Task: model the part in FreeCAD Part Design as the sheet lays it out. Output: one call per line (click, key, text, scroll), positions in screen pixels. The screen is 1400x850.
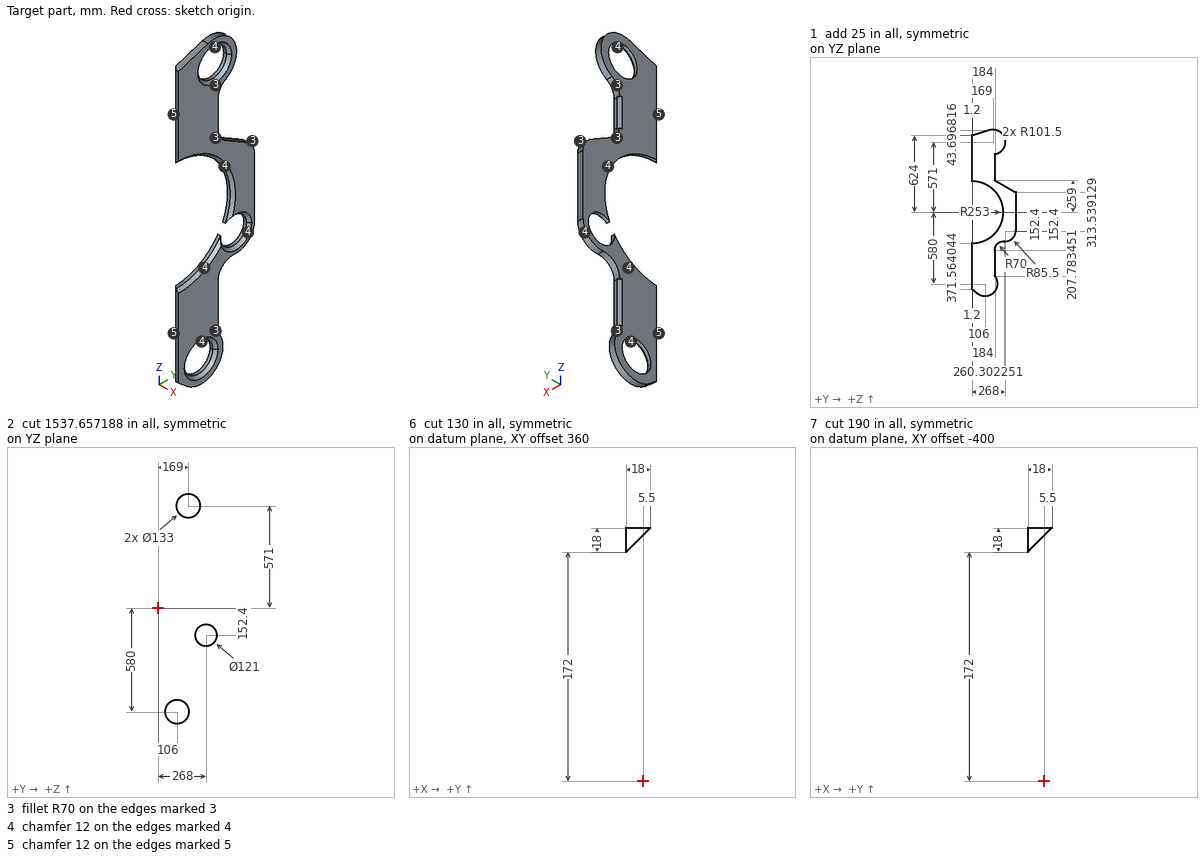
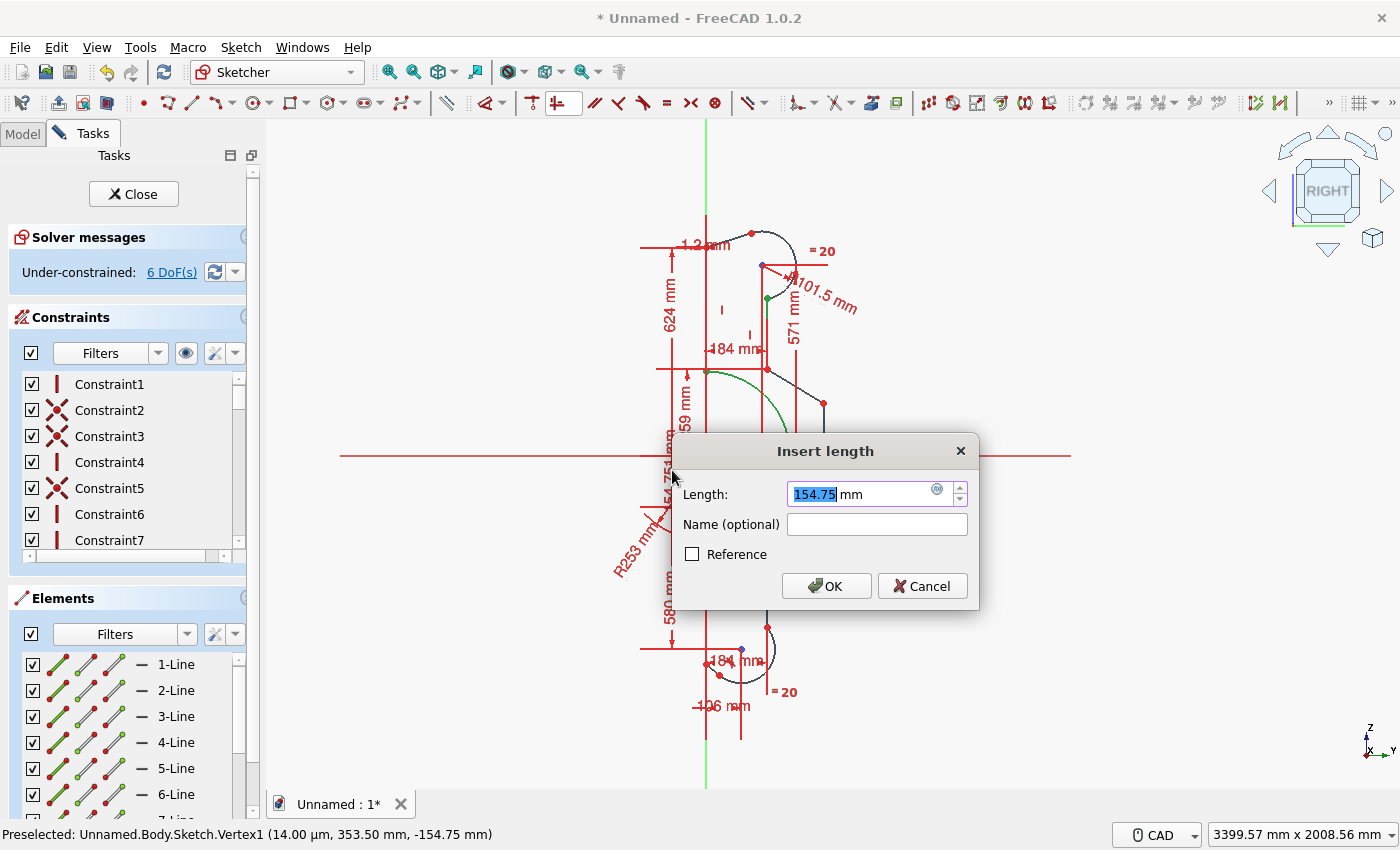
text(152.4)
key(Return)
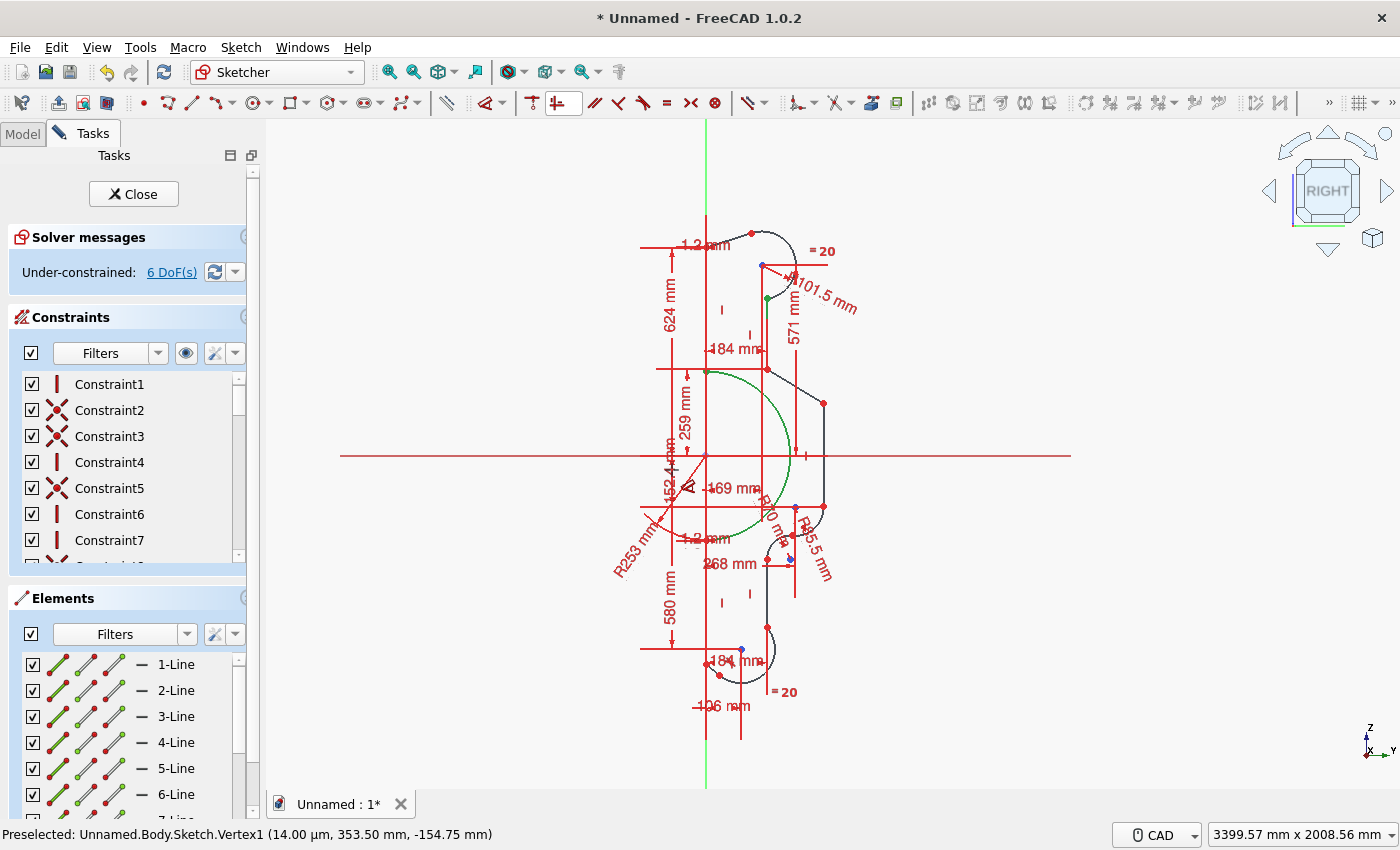
click(795, 507)
click(648, 493)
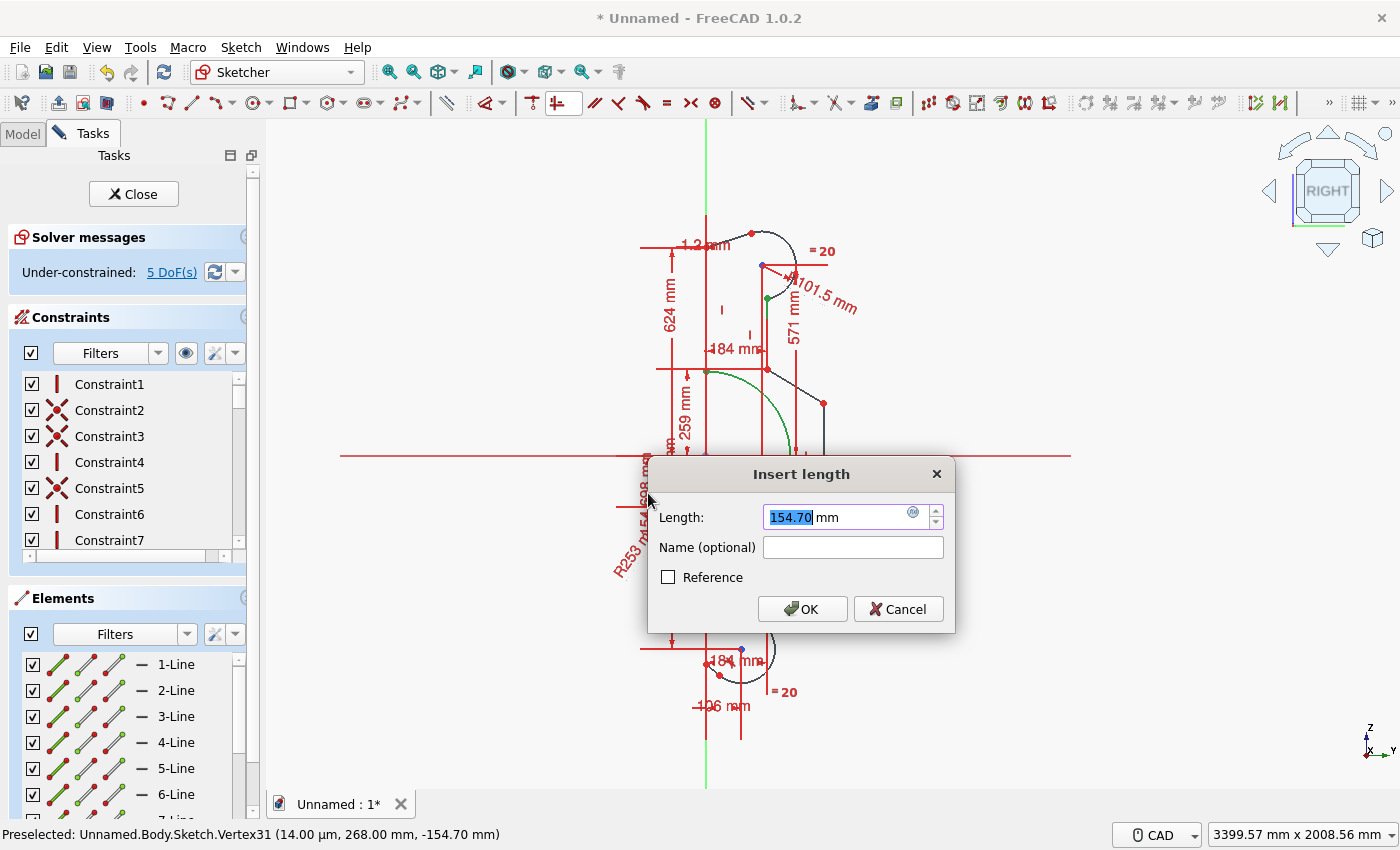
text(152.4)
key(Return)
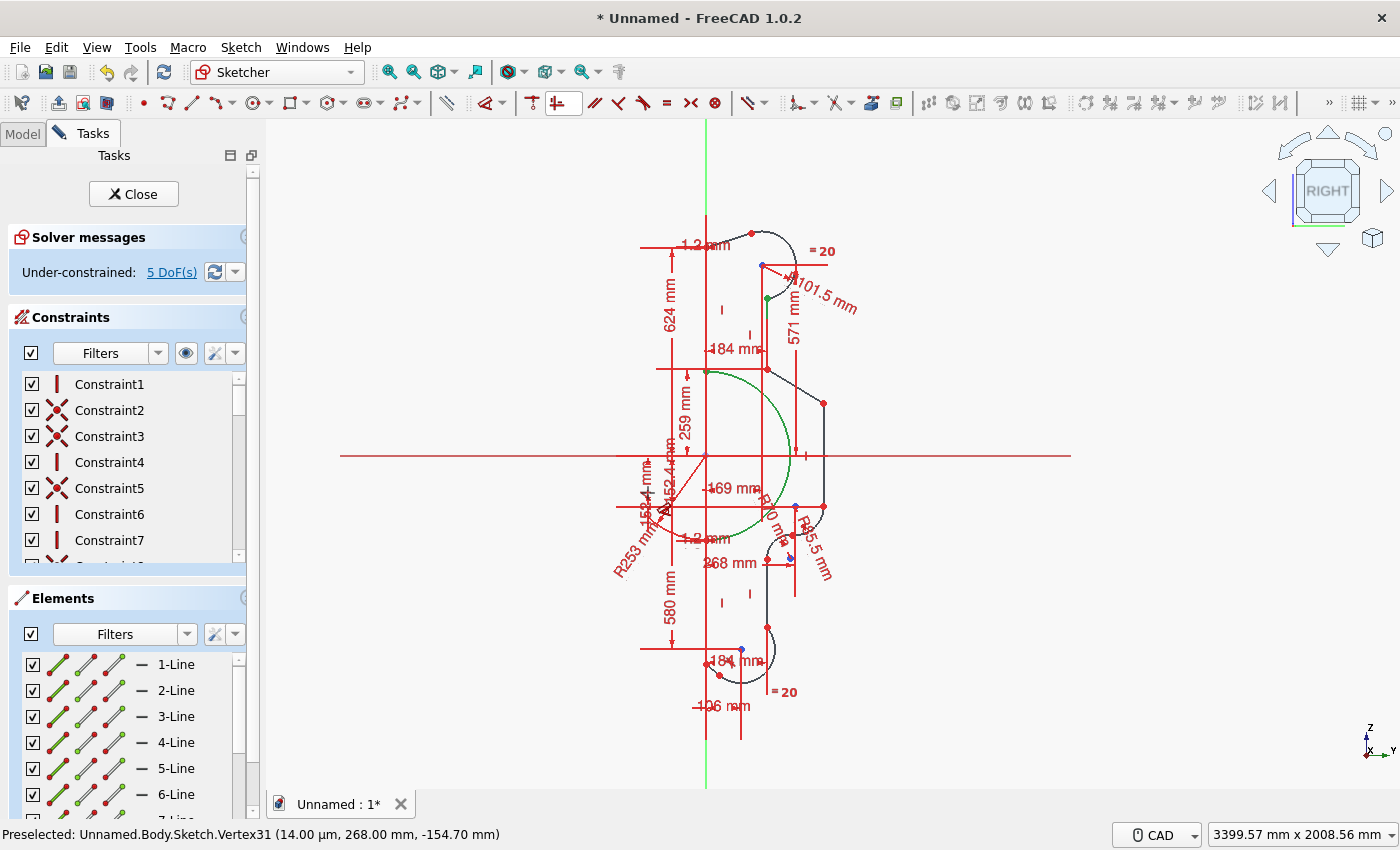
click(824, 476)
click(858, 431)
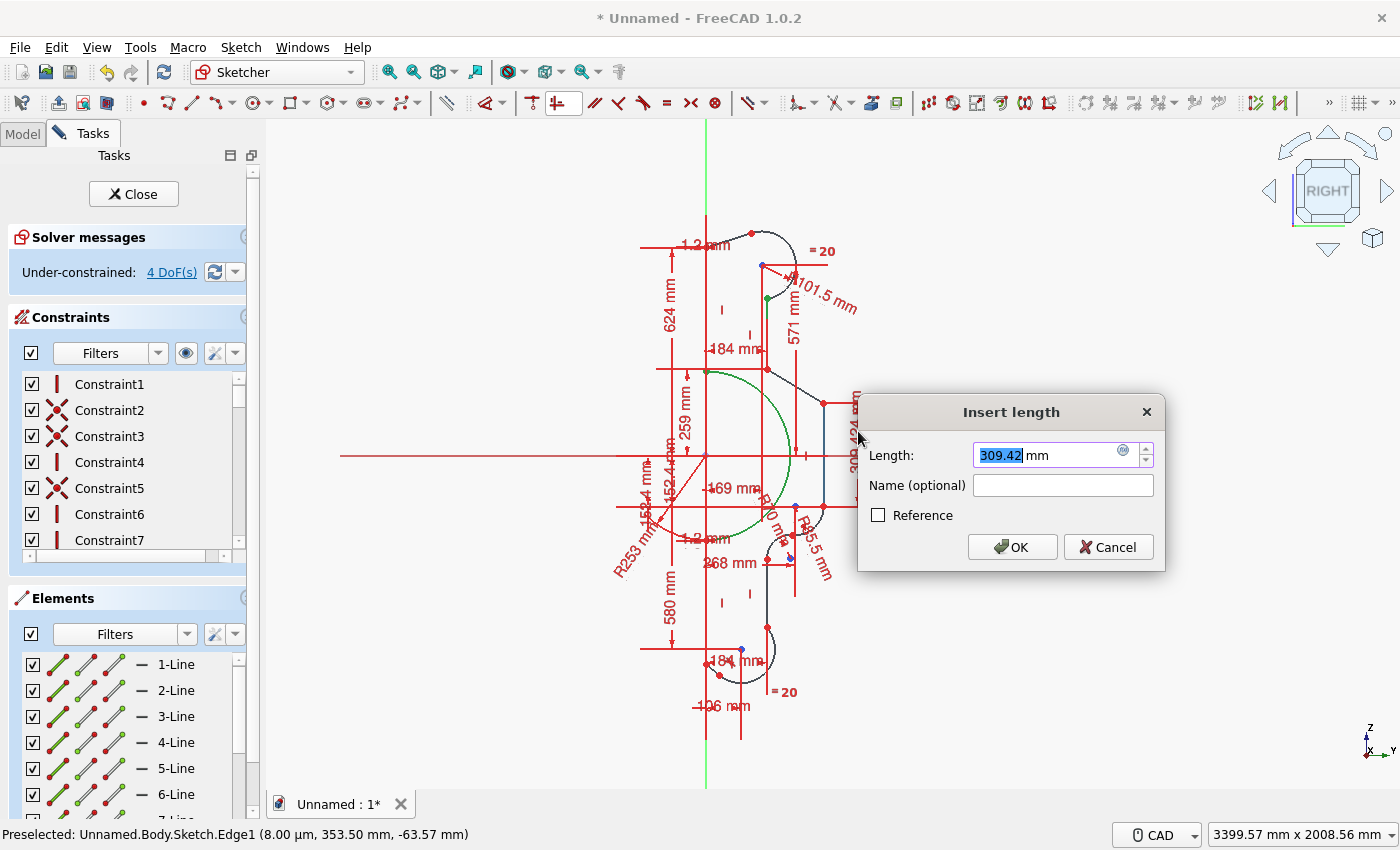
text(313.539129)
key(Return)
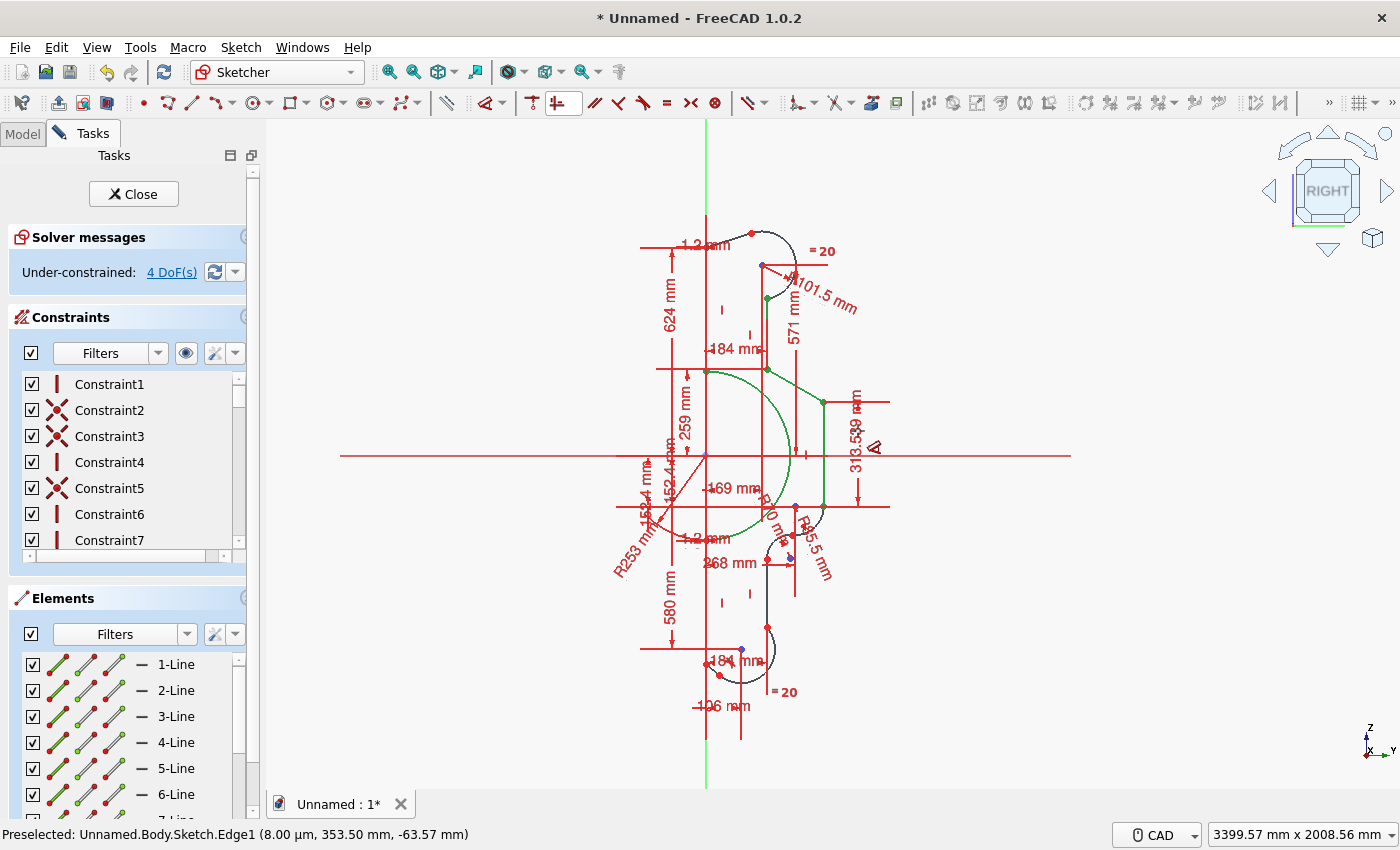
click(706, 577)
click(672, 631)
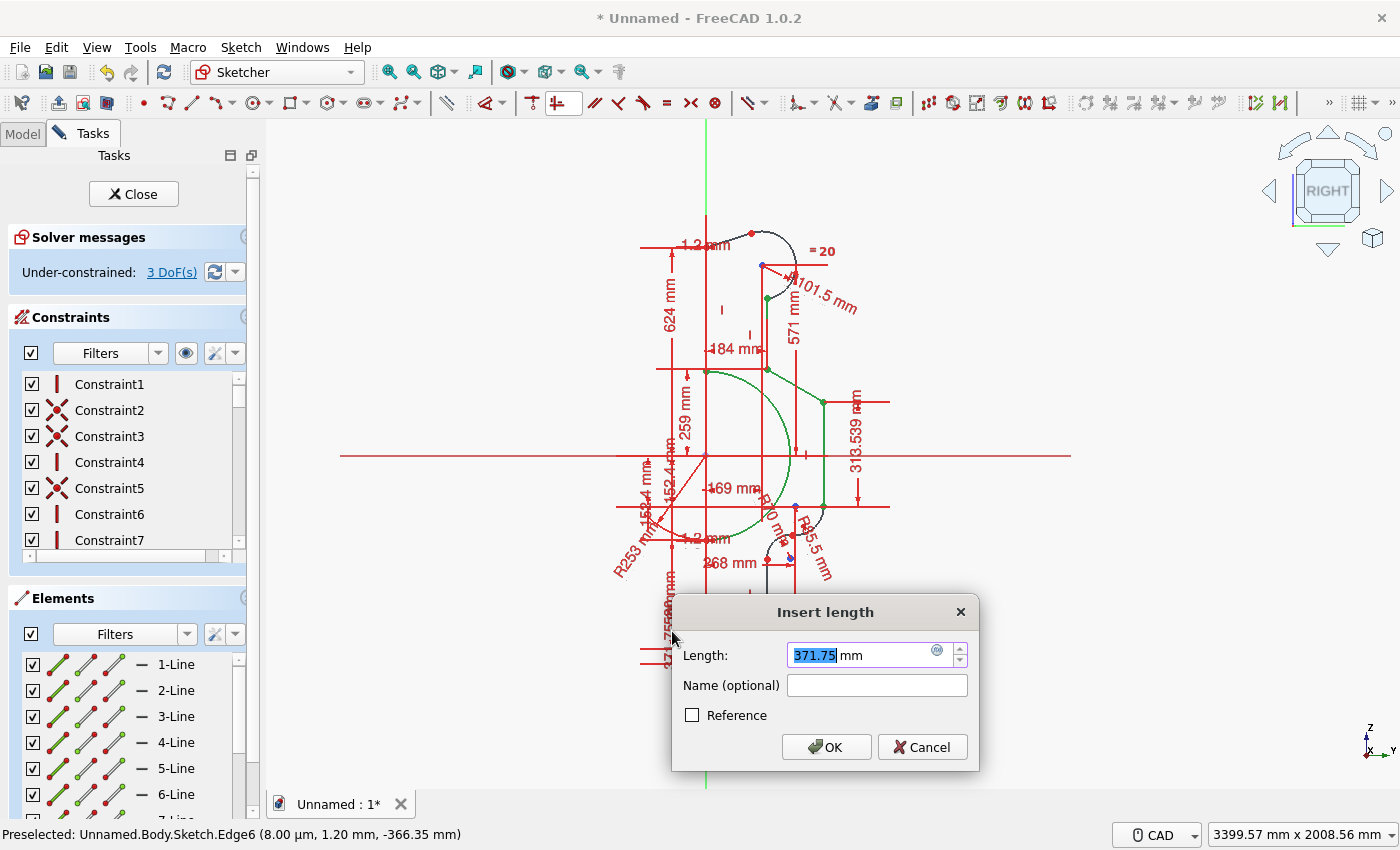
text(371.564044)
key(Return)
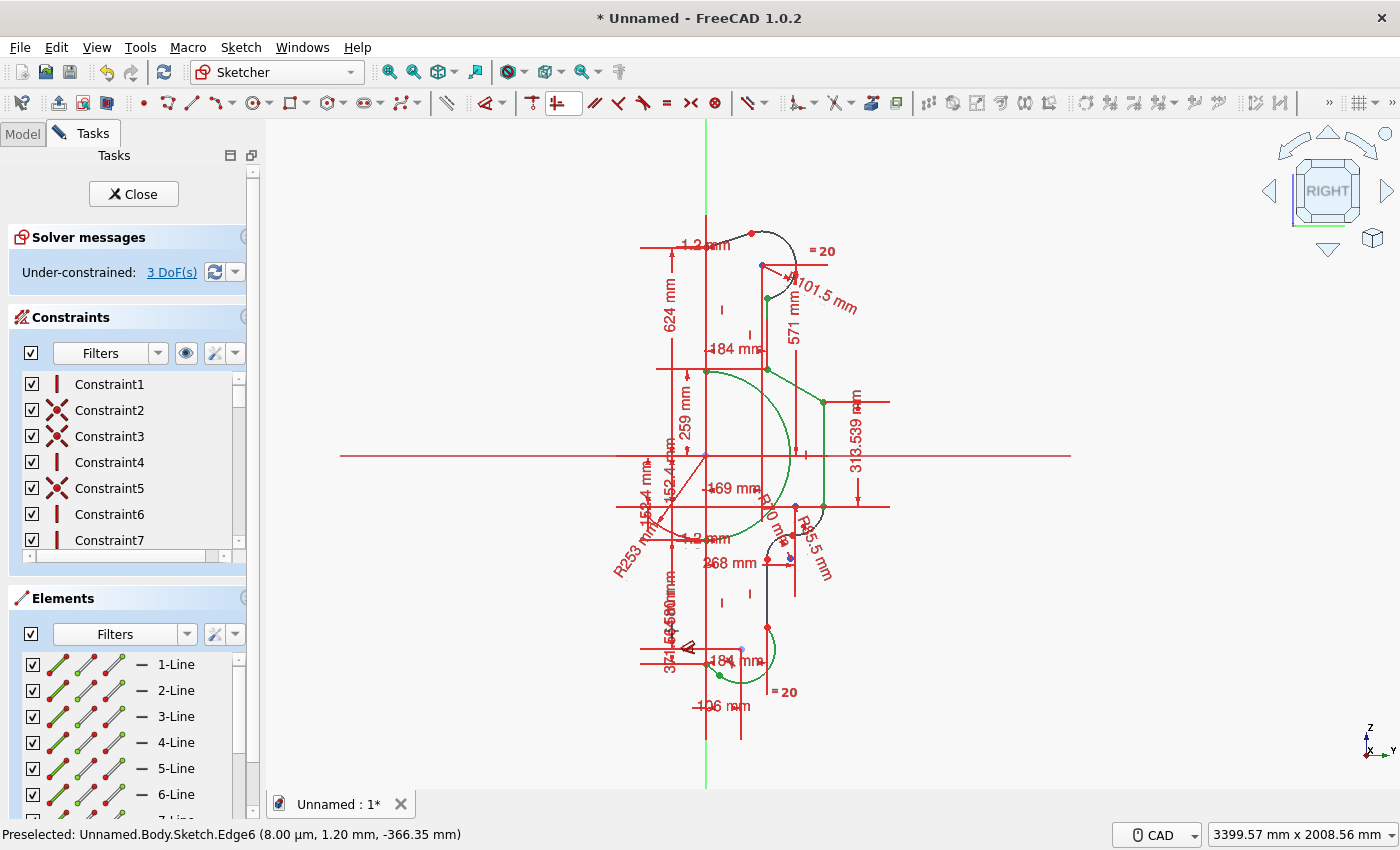
click(767, 607)
click(801, 593)